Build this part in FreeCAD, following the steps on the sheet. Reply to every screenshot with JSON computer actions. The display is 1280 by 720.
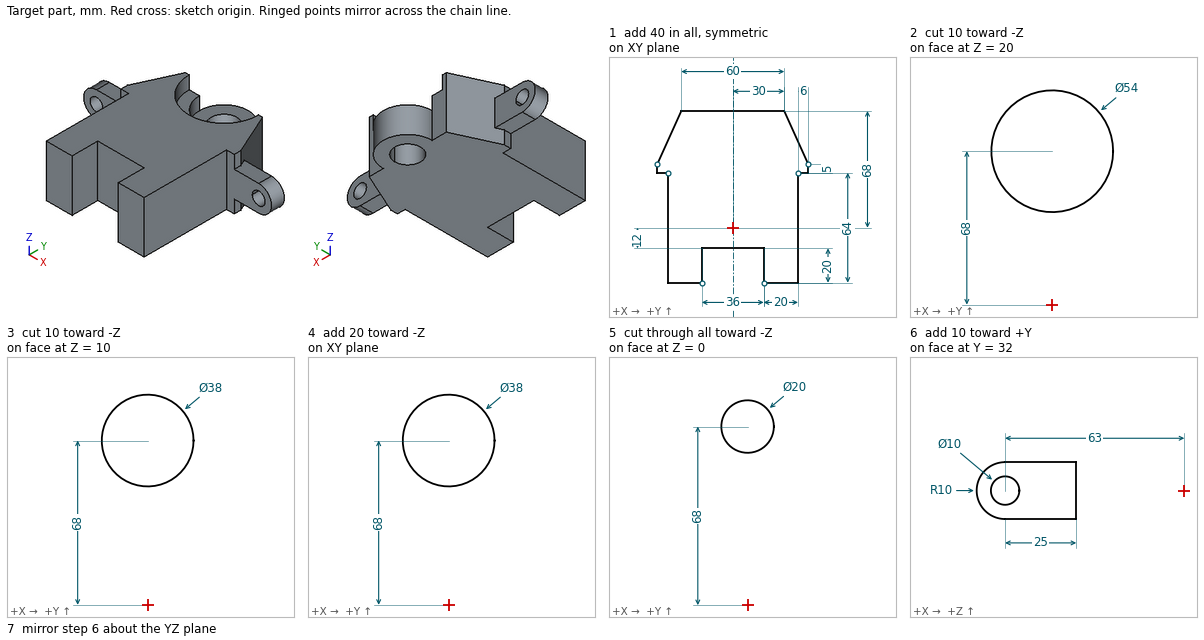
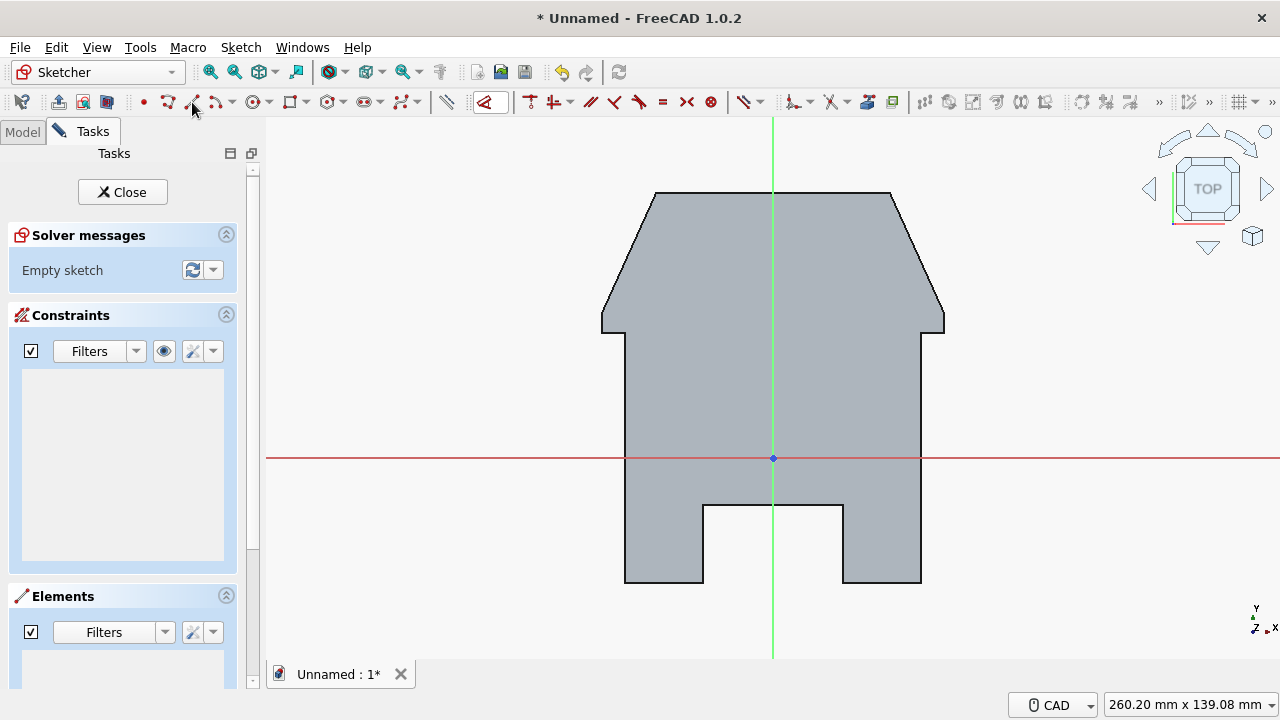
{"action": "scroll", "coordinate": [395, 631], "scroll_direction": "down", "scroll_amount": 1}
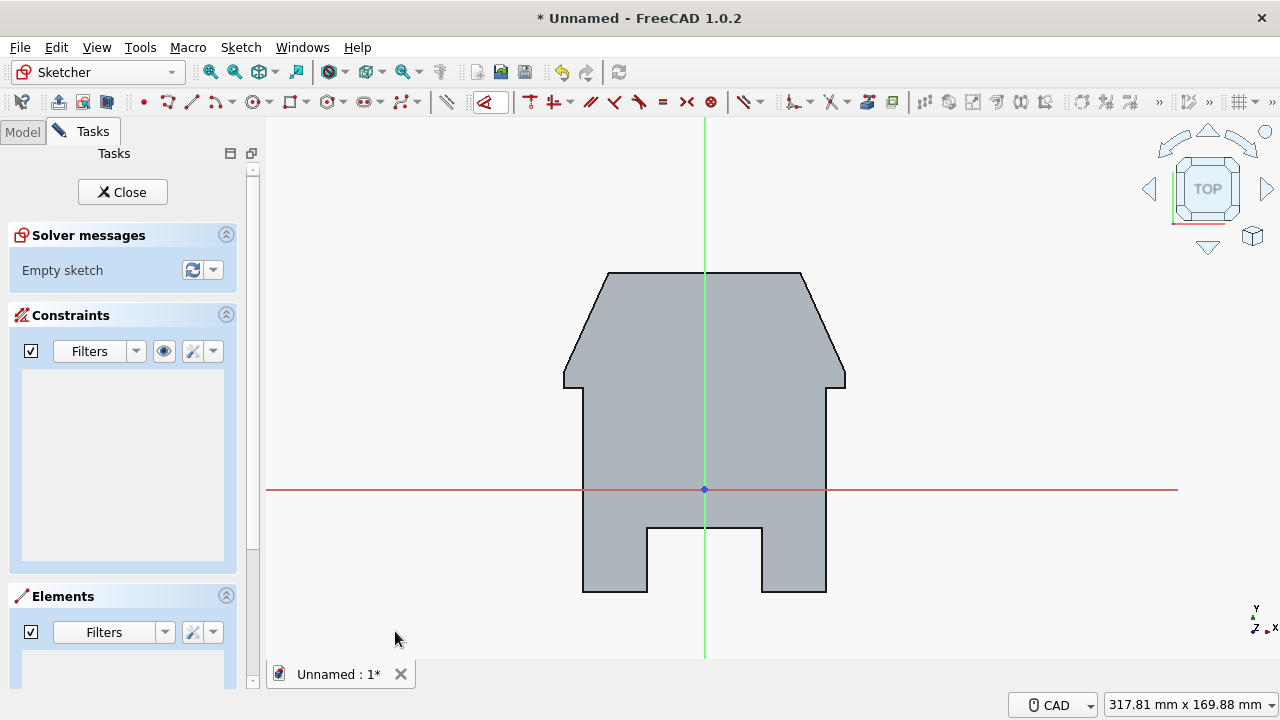
{"action": "left_click", "coordinate": [254, 102]}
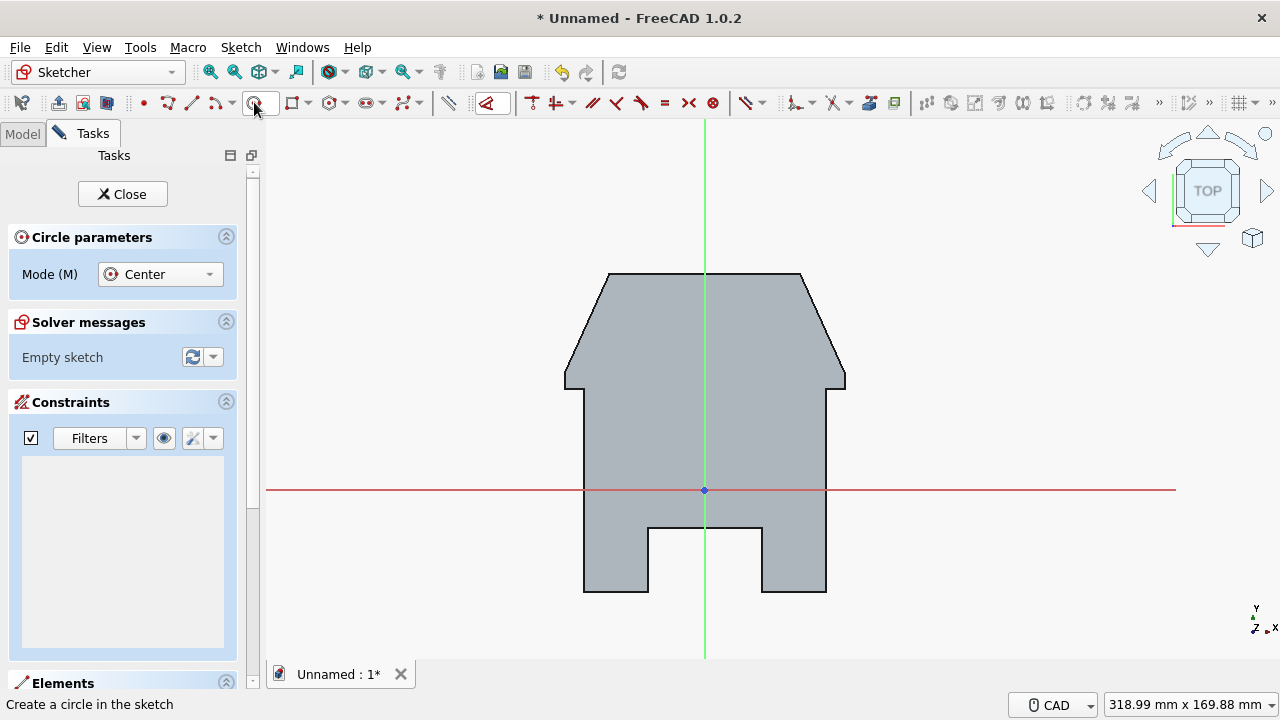
{"action": "left_click", "coordinate": [705, 274]}
{"action": "left_click", "coordinate": [765, 213]}
{"action": "key", "text": "Escape"}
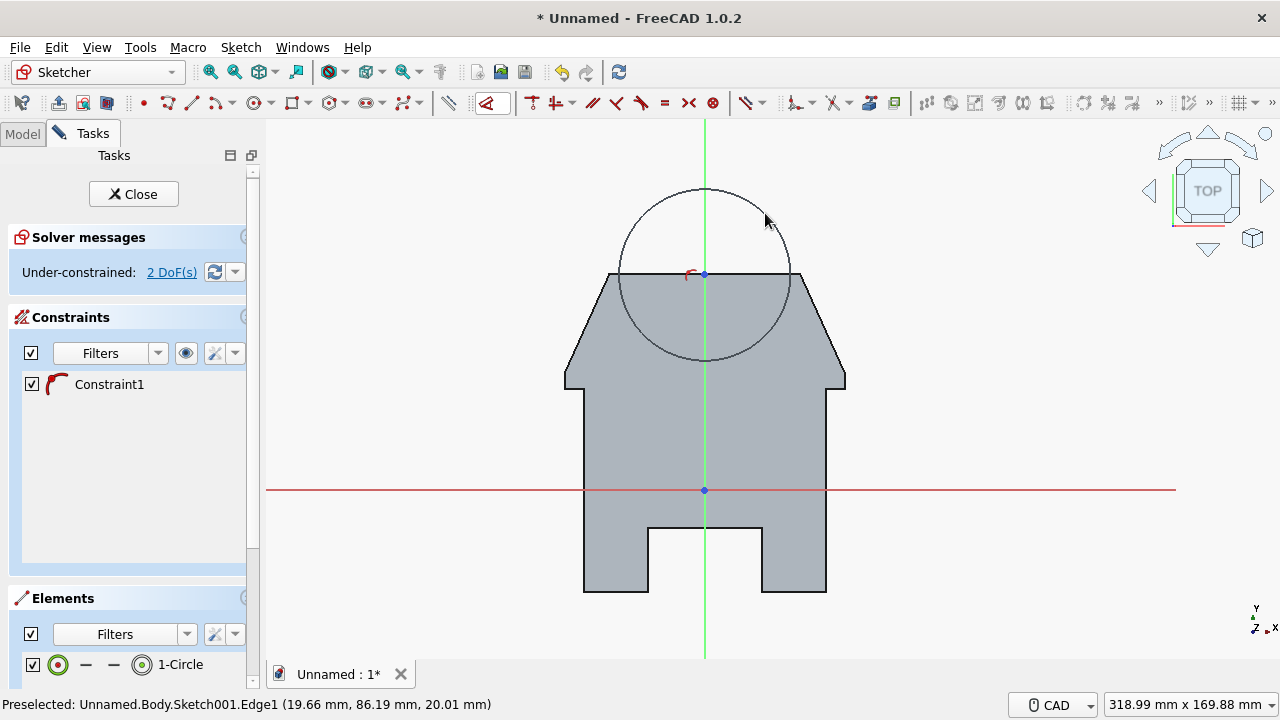
{"action": "left_click", "coordinate": [765, 214]}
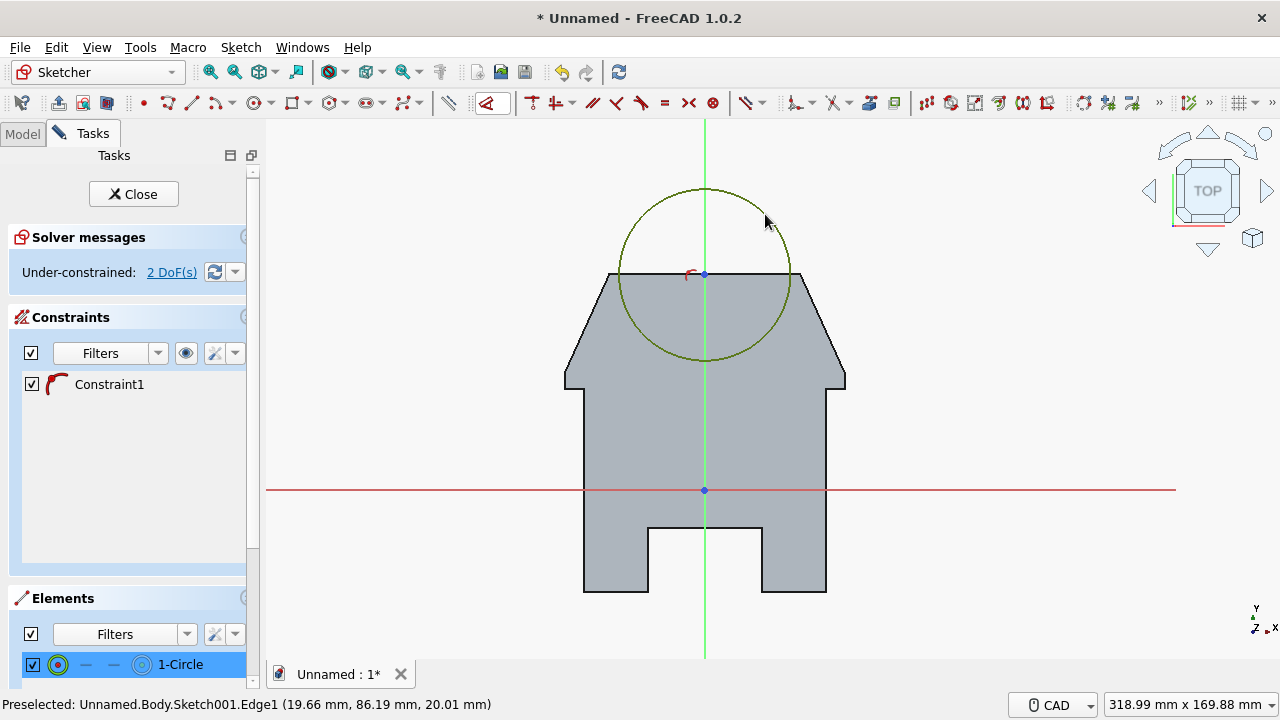
{"action": "key", "text": "k o"}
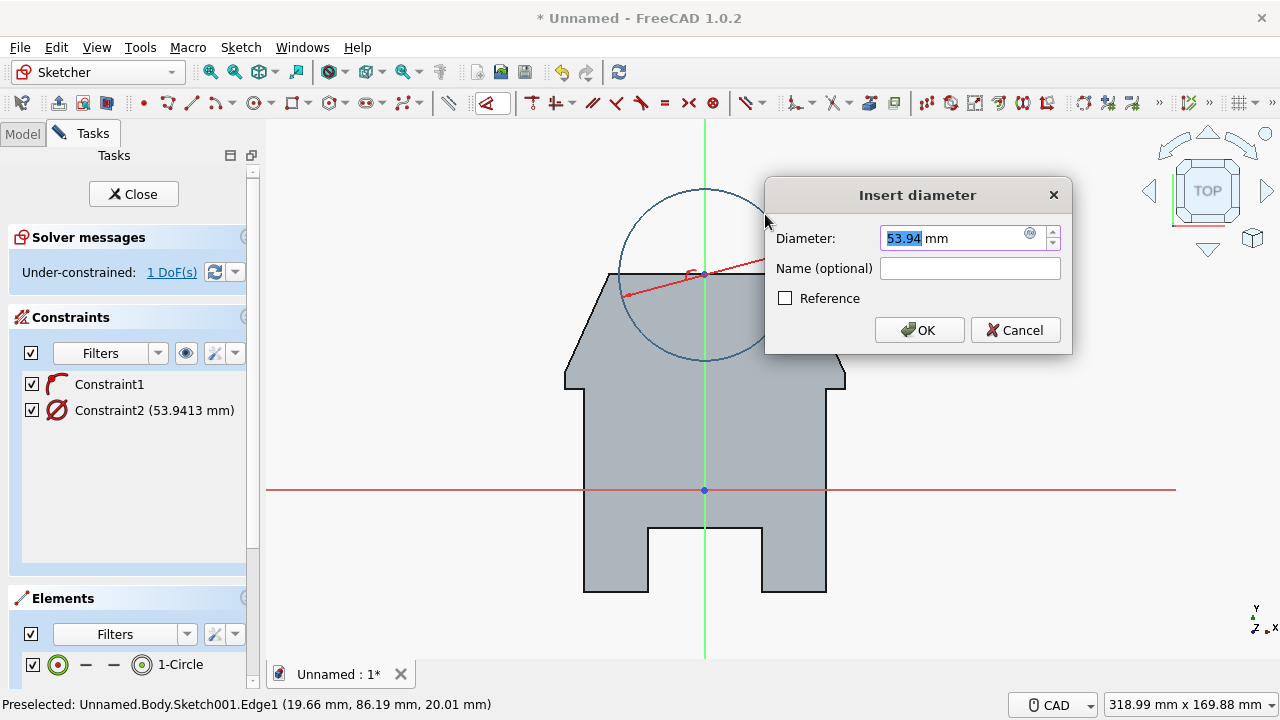
{"action": "type", "text": "54"}
{"action": "key", "text": "Return"}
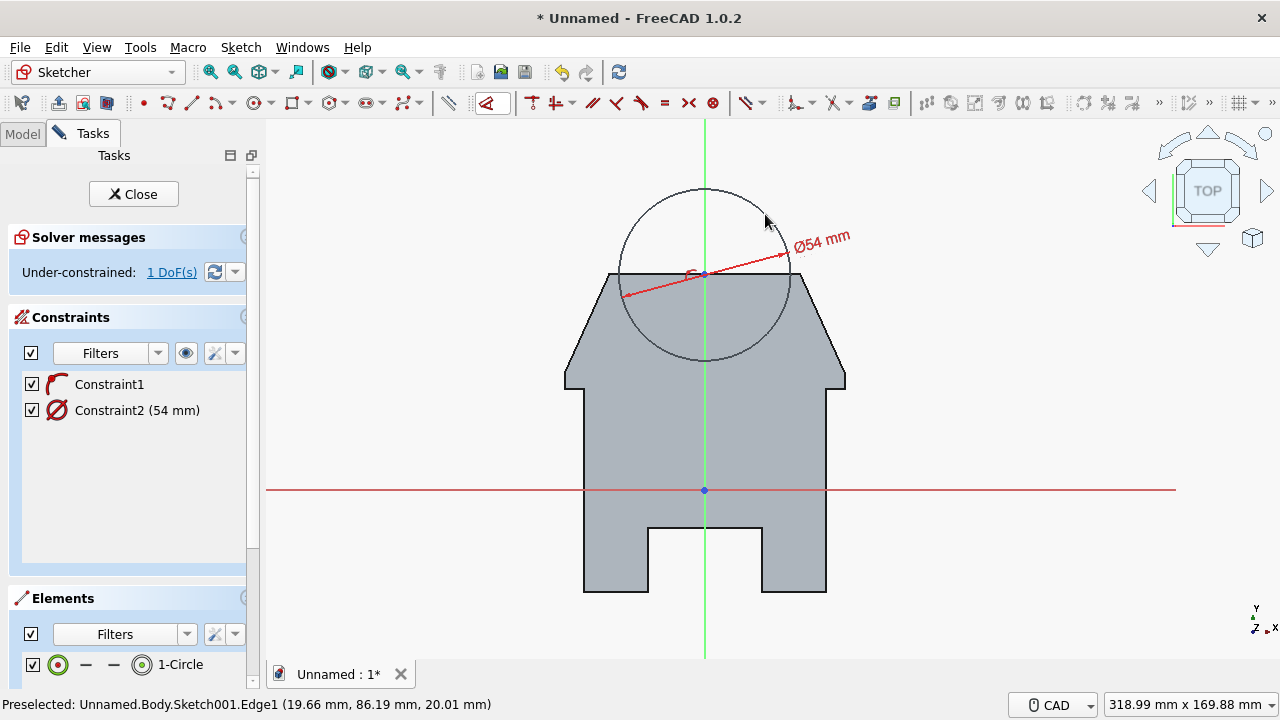
{"action": "left_click", "coordinate": [705, 275]}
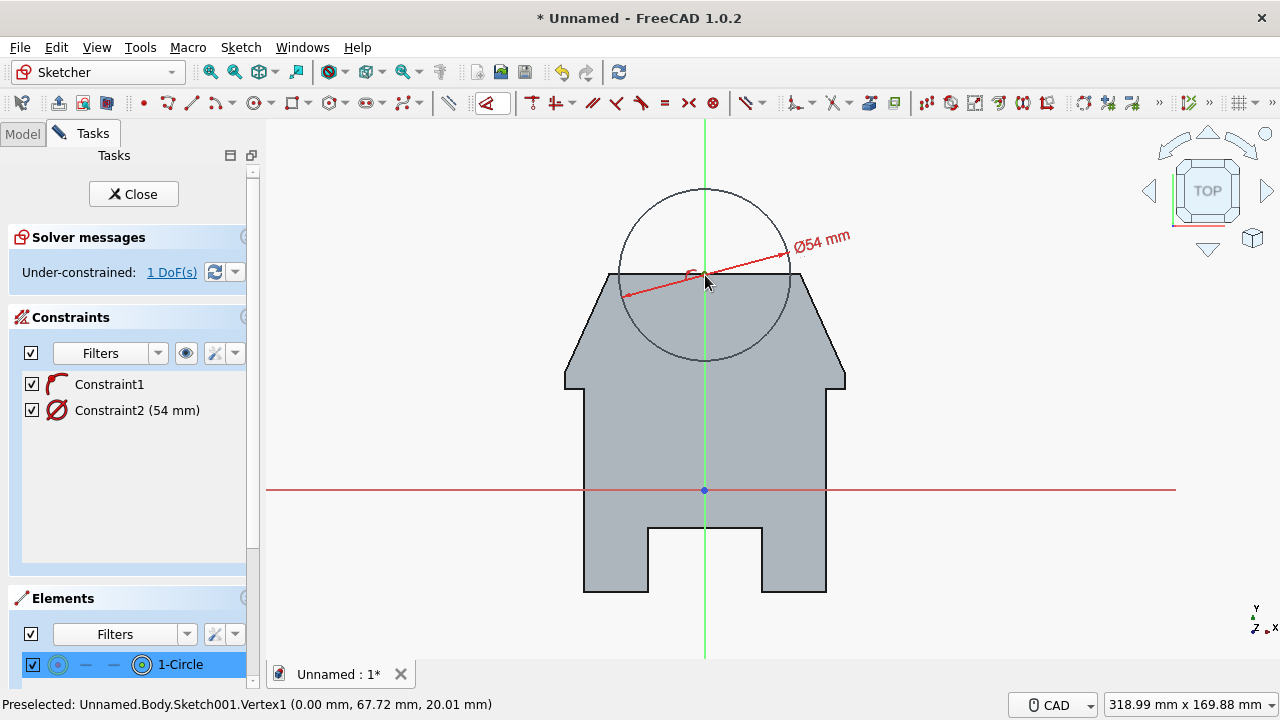
{"action": "left_click", "coordinate": [504, 104]}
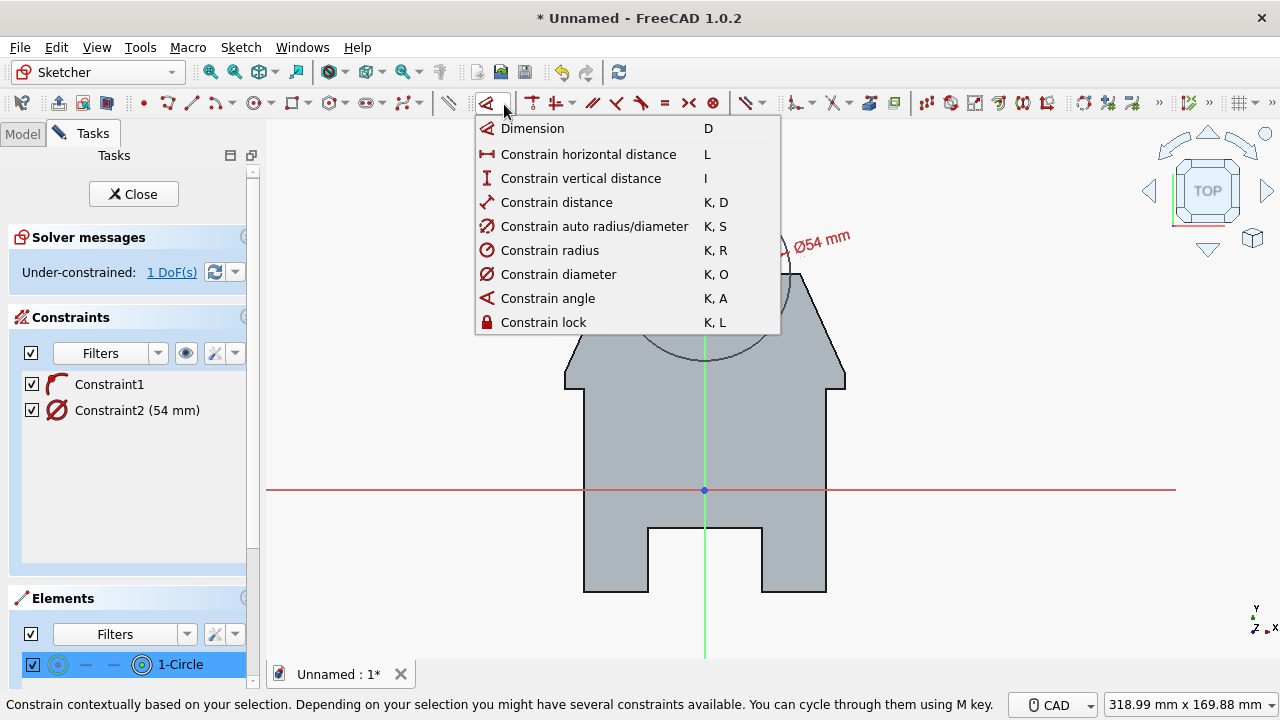
{"action": "left_click", "coordinate": [628, 178]}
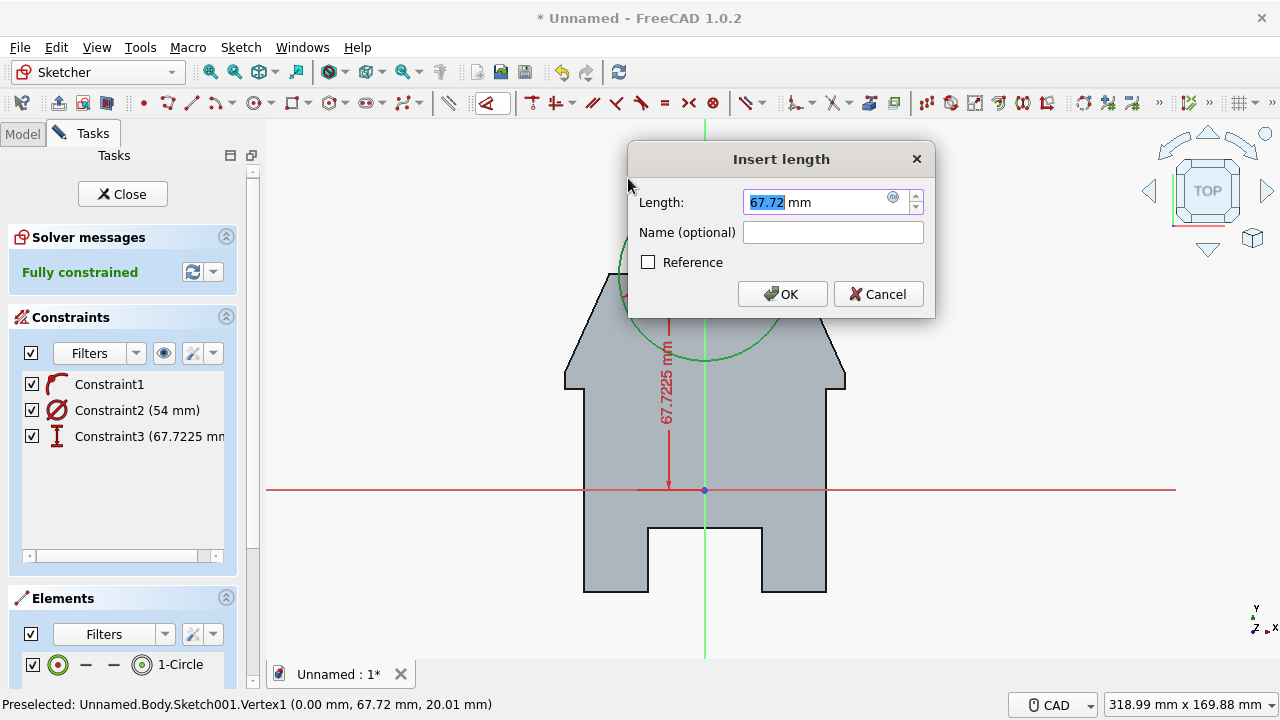
{"action": "type", "text": "68"}
{"action": "key", "text": "Return"}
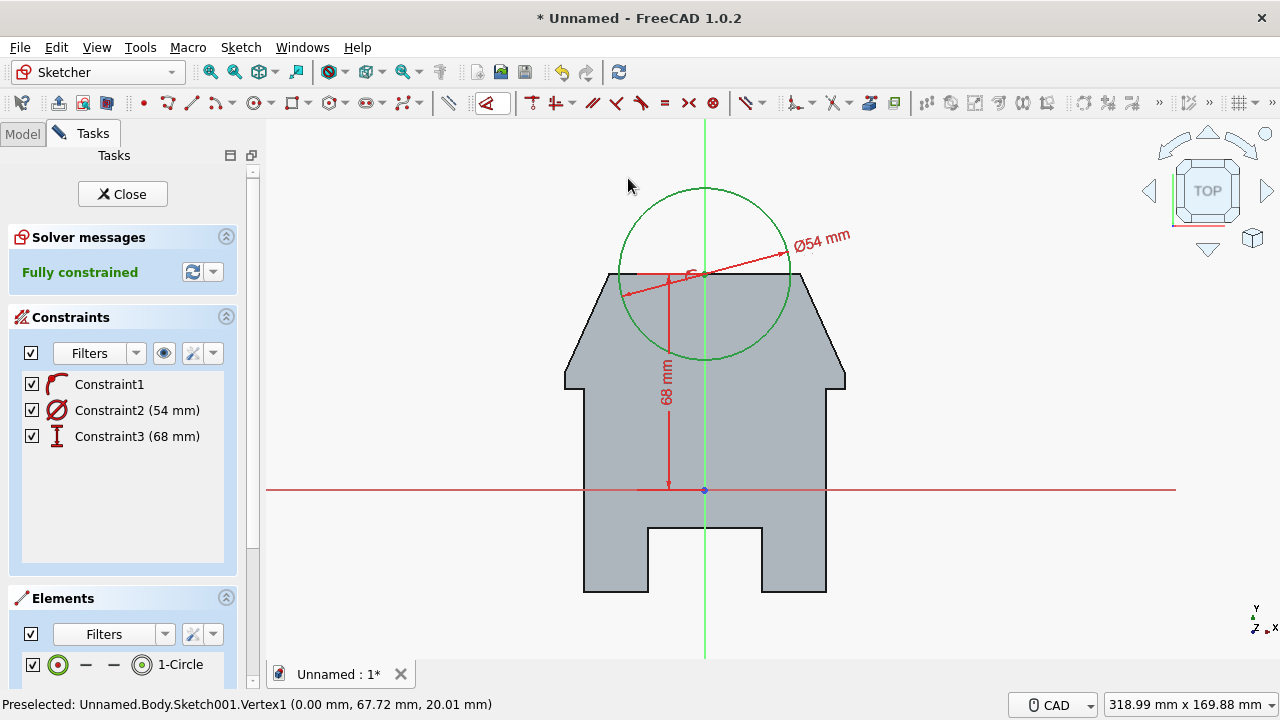
{"action": "left_click", "coordinate": [123, 194]}